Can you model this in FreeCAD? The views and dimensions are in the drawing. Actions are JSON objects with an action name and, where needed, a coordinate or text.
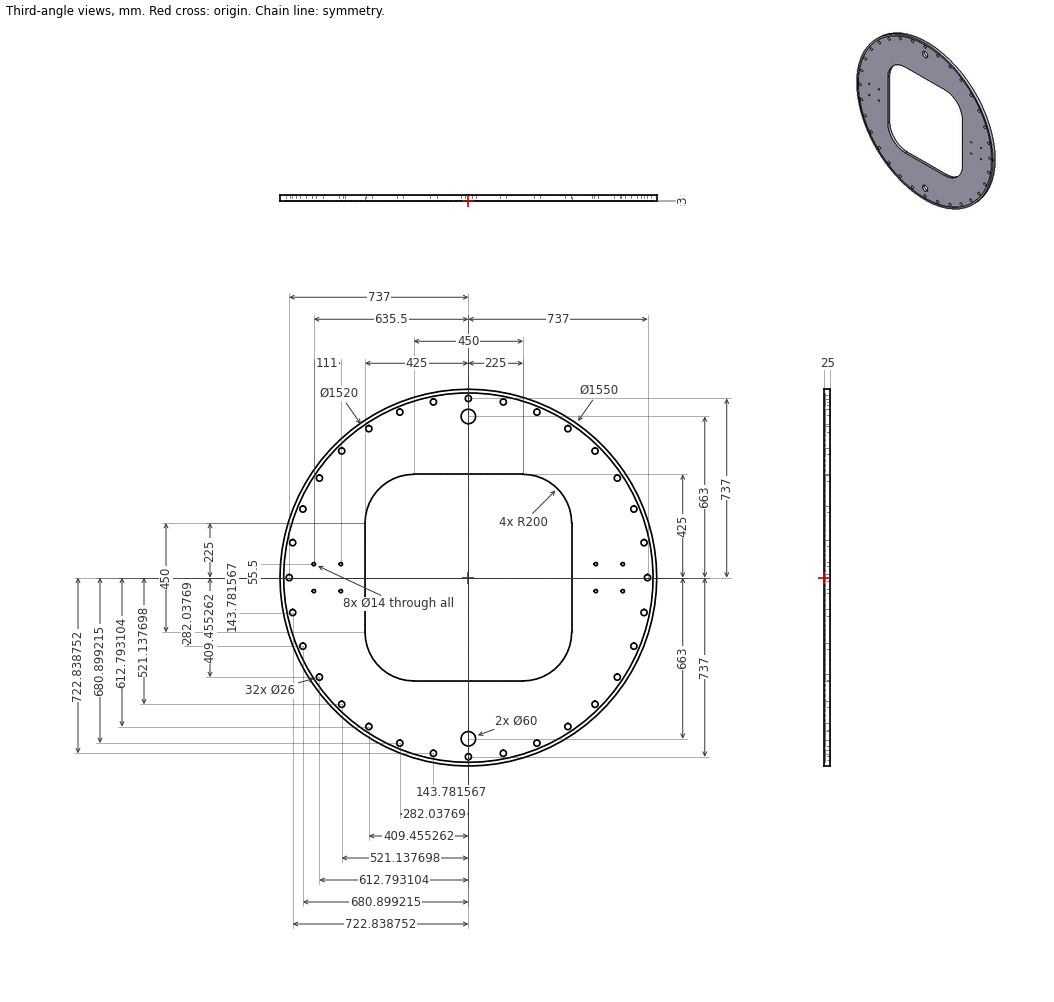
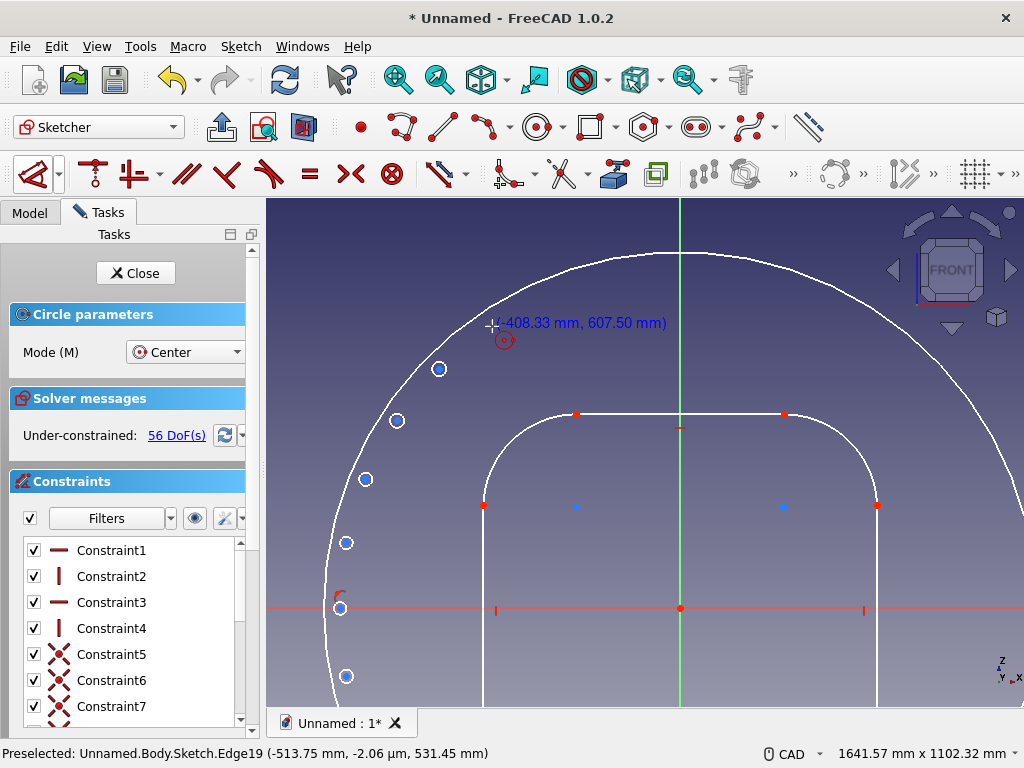
{"action": "left_click", "coordinate": [491, 325]}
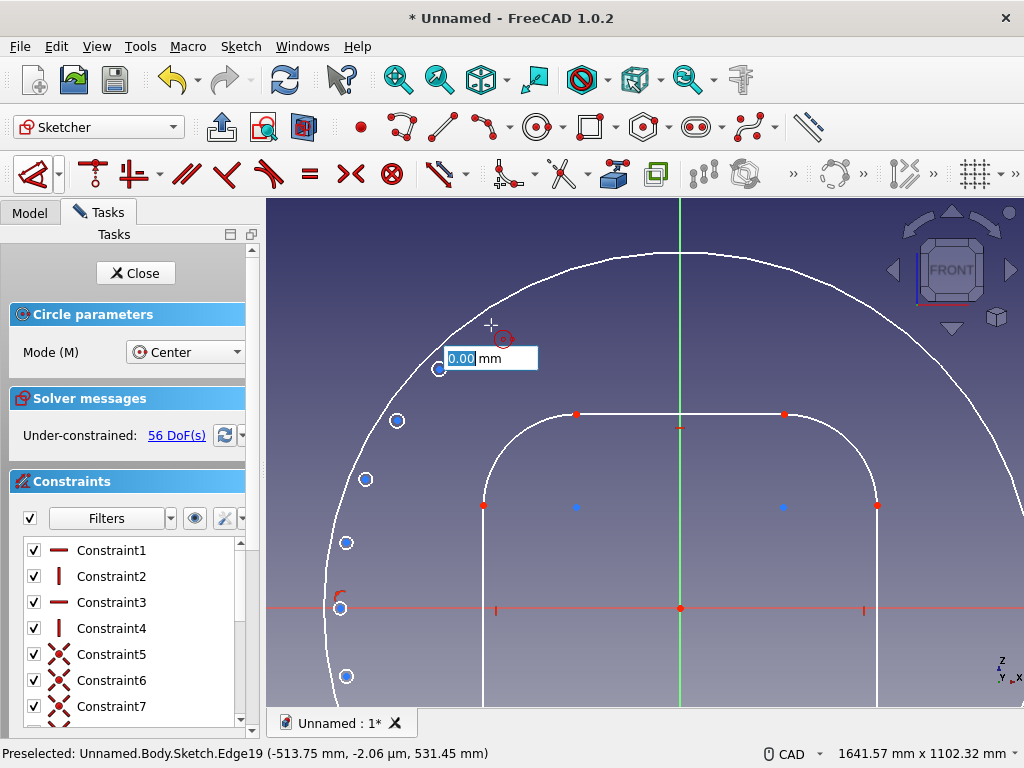
{"action": "scroll", "coordinate": [495, 321], "scroll_direction": "up", "scroll_amount": 5}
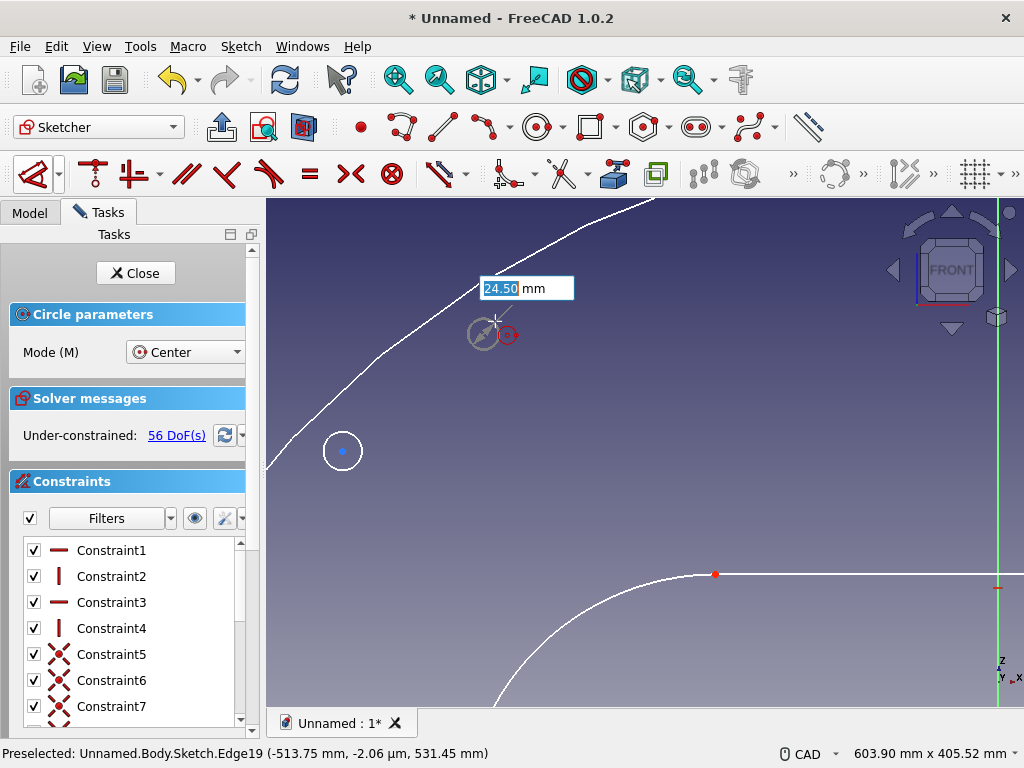
{"action": "left_click", "coordinate": [495, 321]}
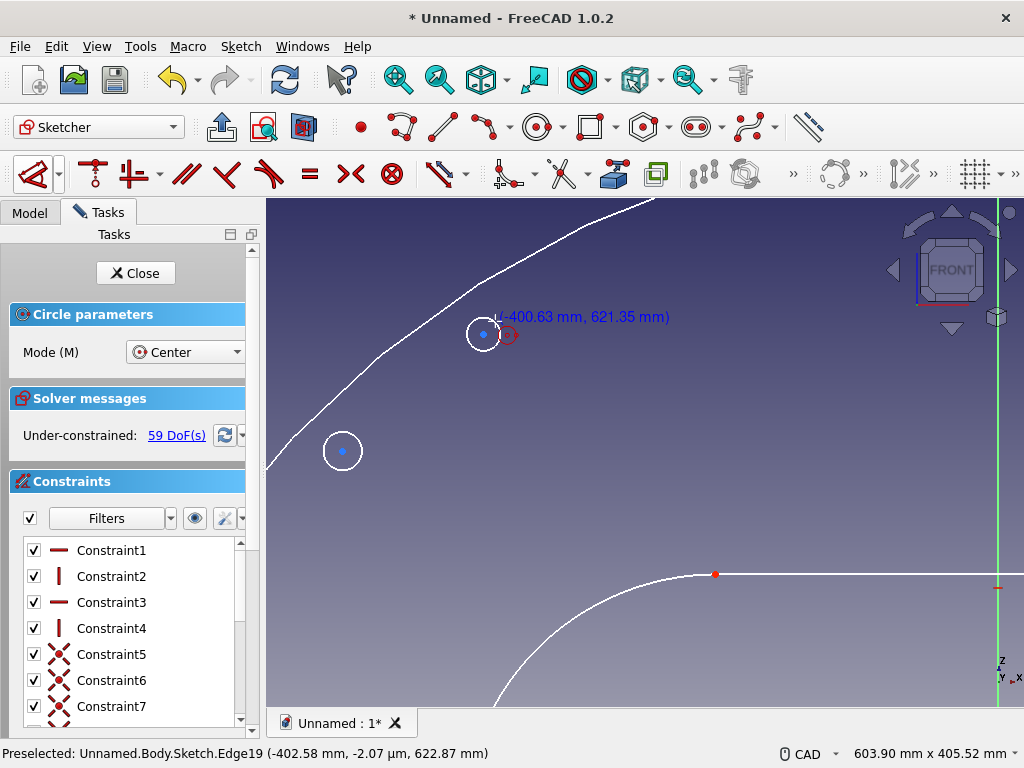
{"action": "scroll", "coordinate": [644, 247], "scroll_direction": "up", "scroll_amount": 2}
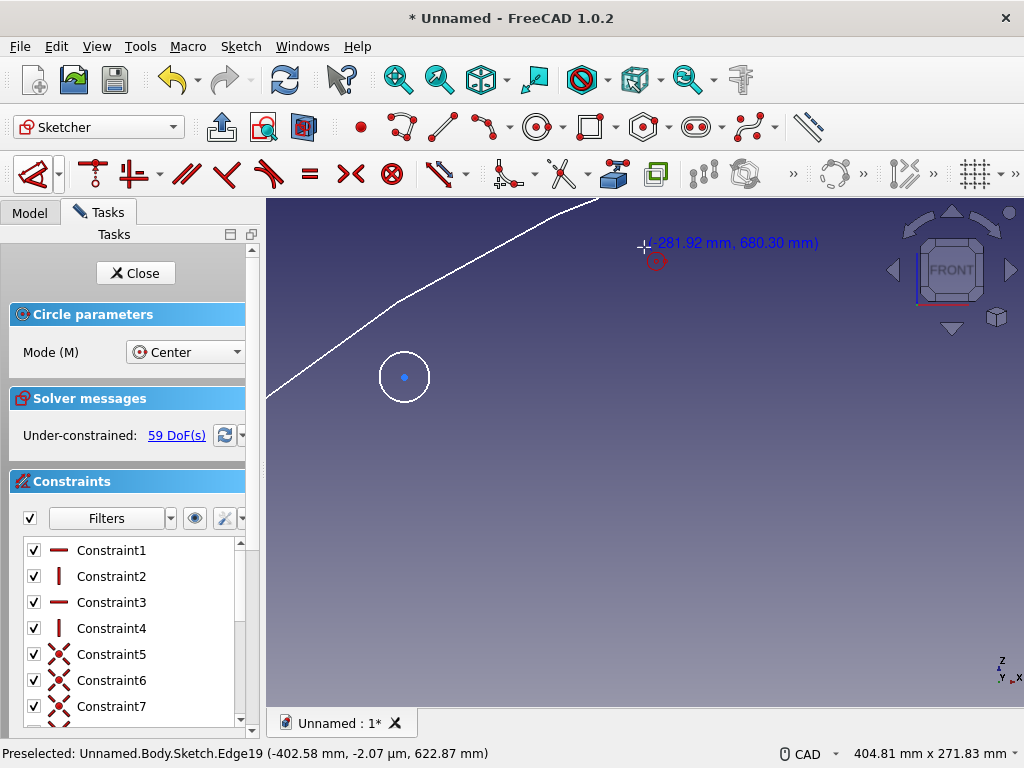
{"action": "scroll", "coordinate": [502, 319], "scroll_direction": "down", "scroll_amount": 11}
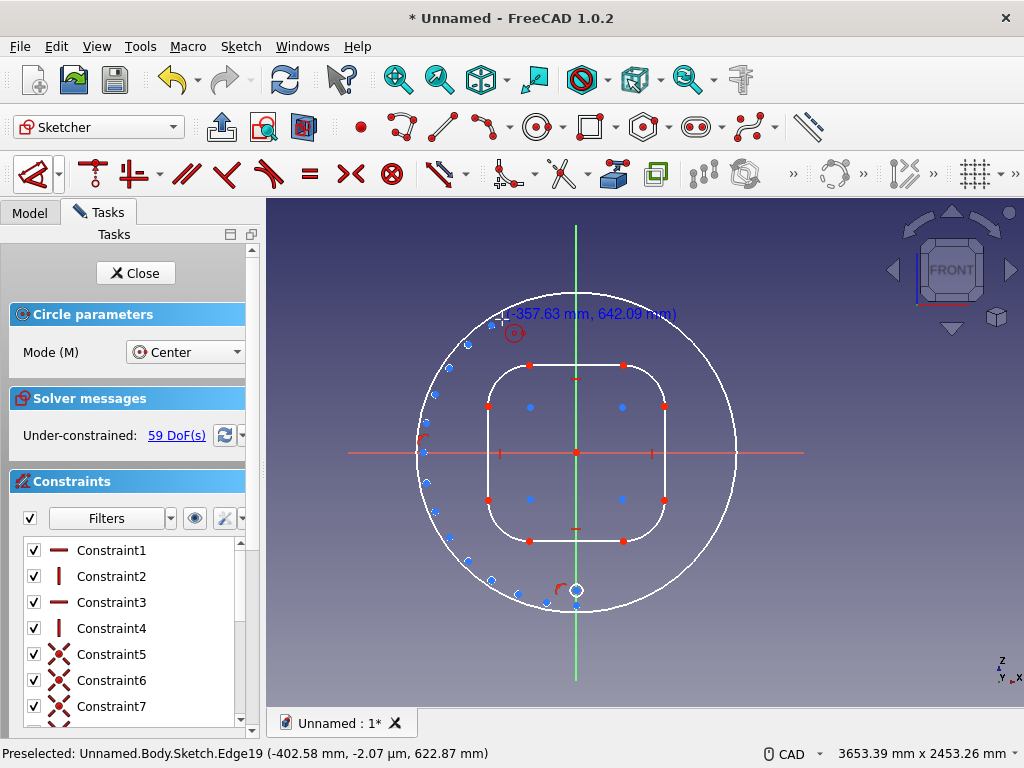
{"action": "scroll", "coordinate": [518, 311], "scroll_direction": "up", "scroll_amount": 4}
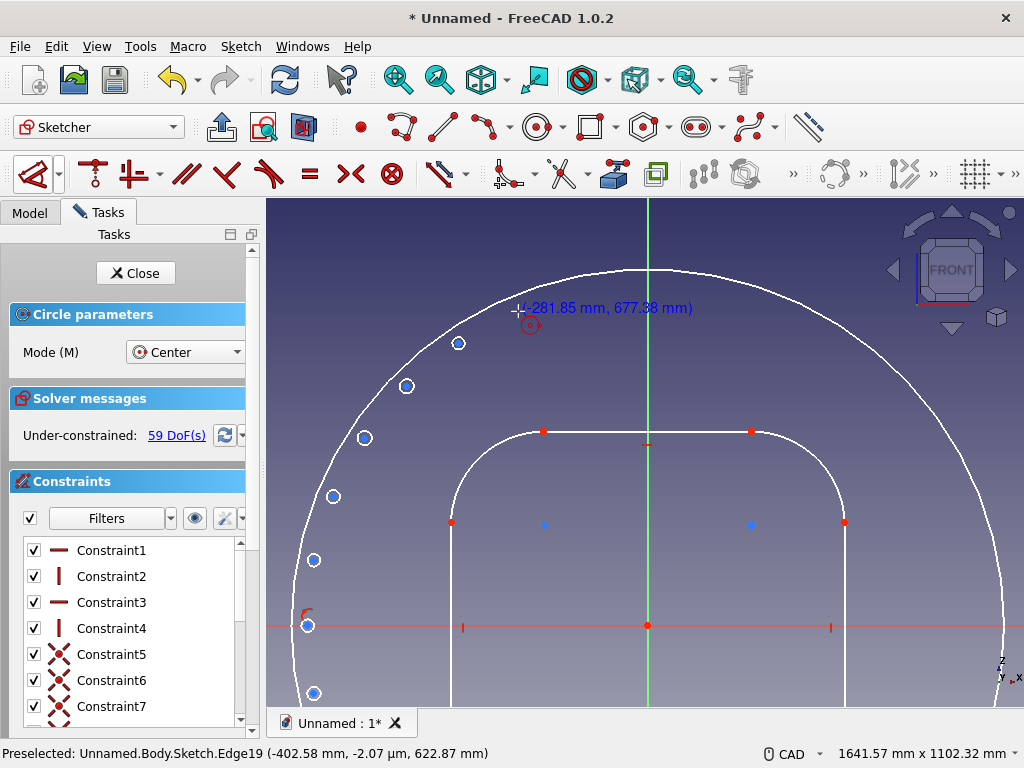
{"action": "left_click", "coordinate": [518, 311]}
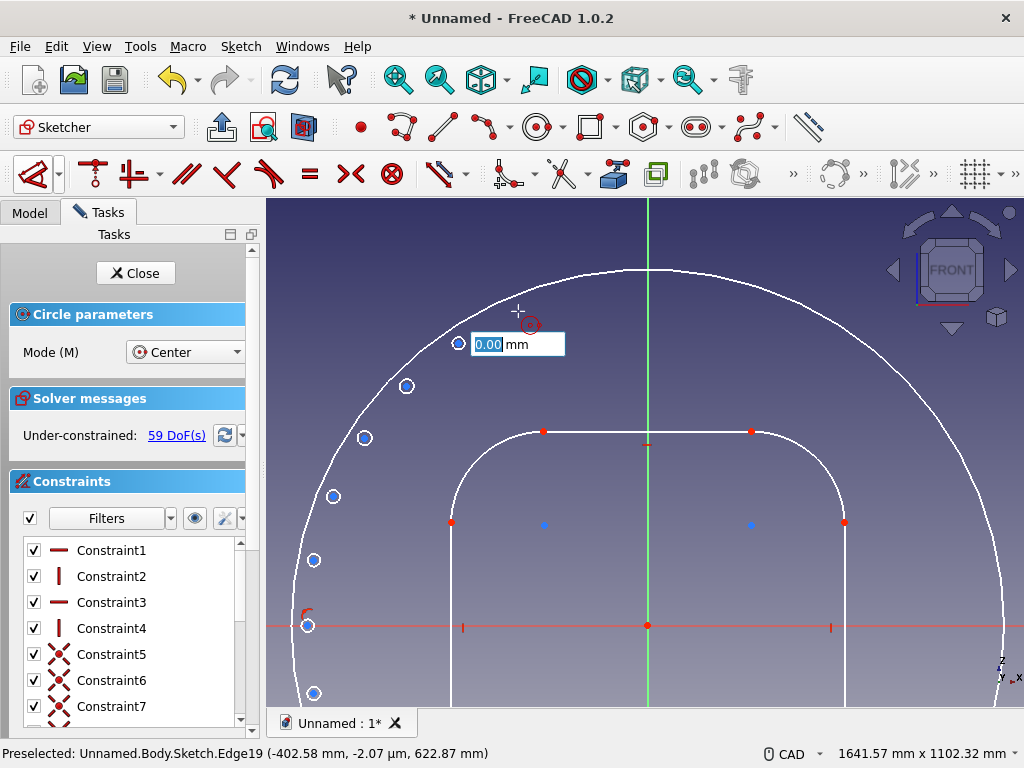
{"action": "scroll", "coordinate": [522, 307], "scroll_direction": "up", "scroll_amount": 5}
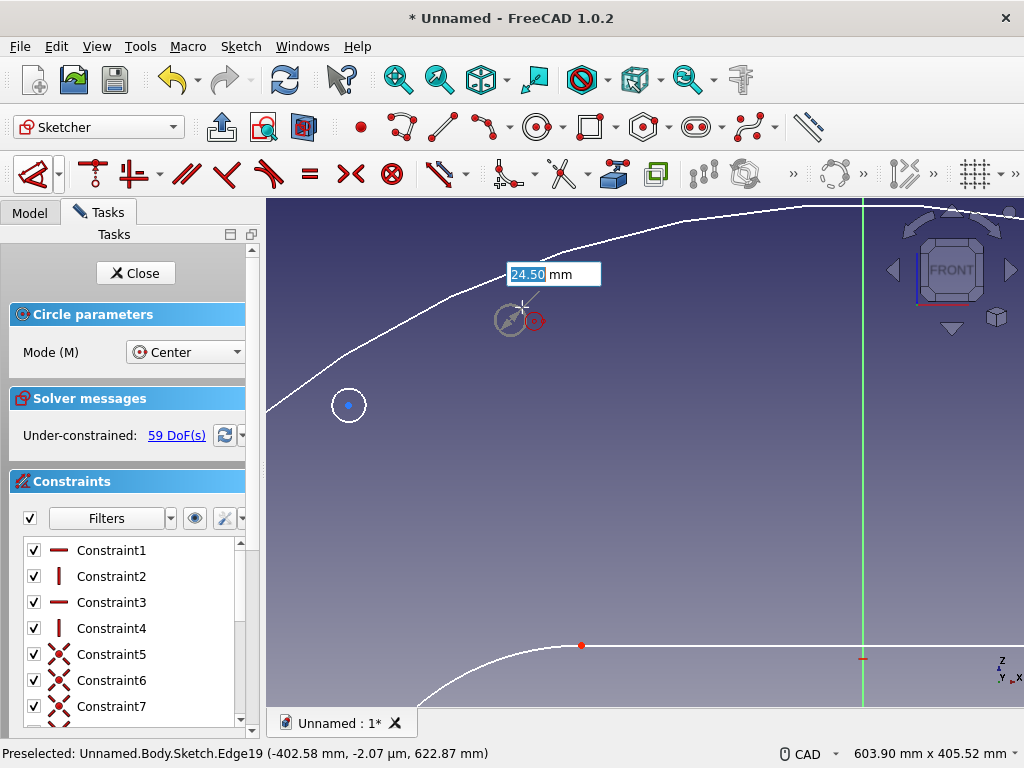
{"action": "left_click", "coordinate": [521, 307]}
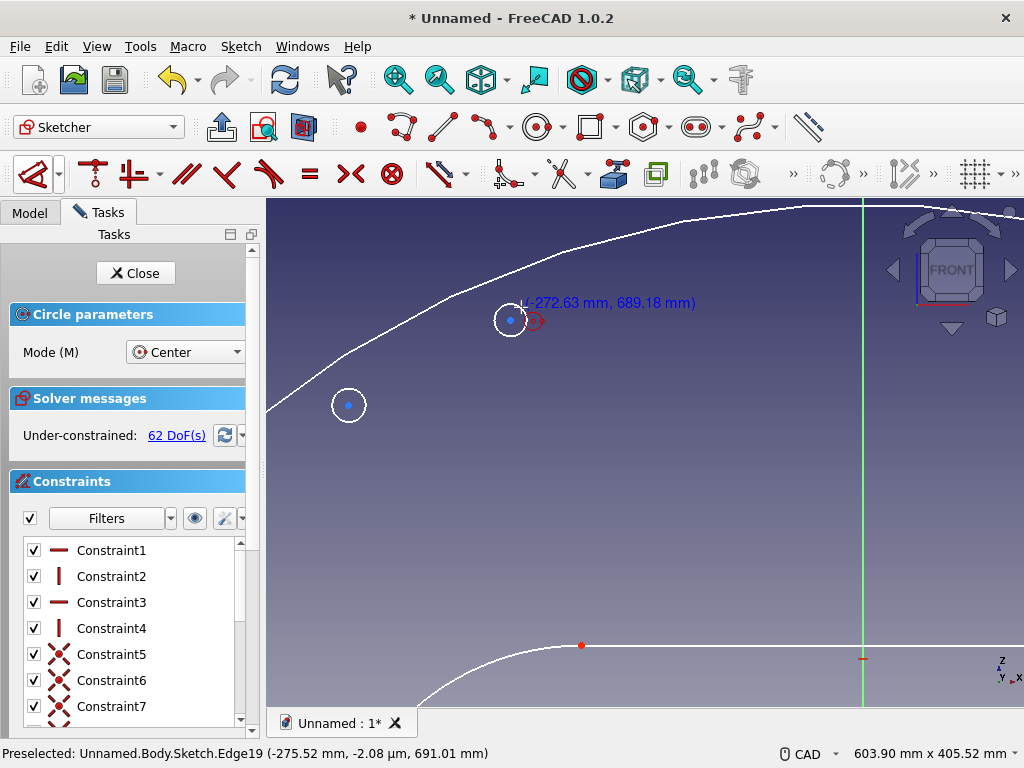
{"action": "scroll", "coordinate": [683, 266], "scroll_direction": "up", "scroll_amount": 2}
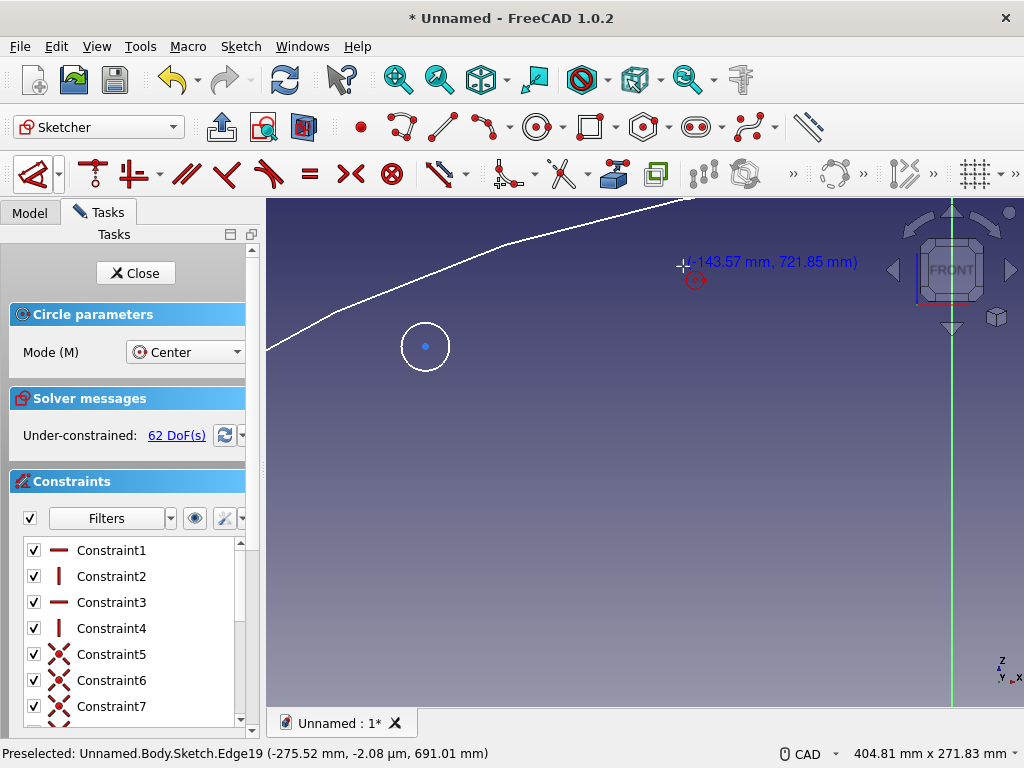
{"action": "scroll", "coordinate": [530, 307], "scroll_direction": "down", "scroll_amount": 11}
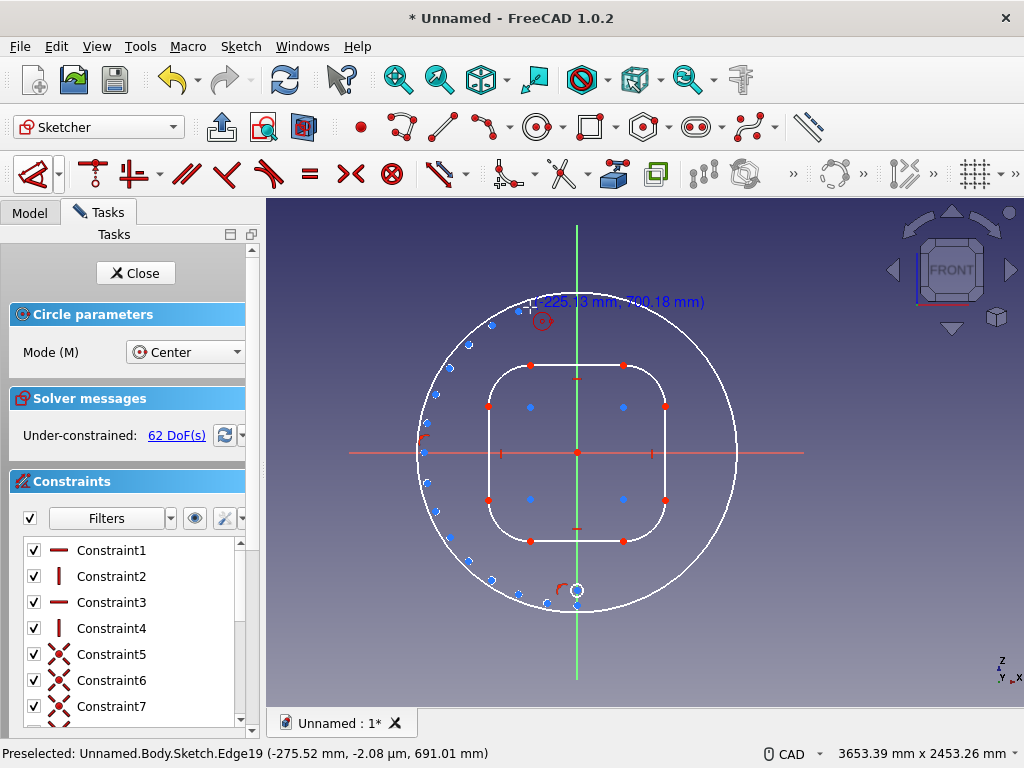
{"action": "scroll", "coordinate": [547, 303], "scroll_direction": "up", "scroll_amount": 4}